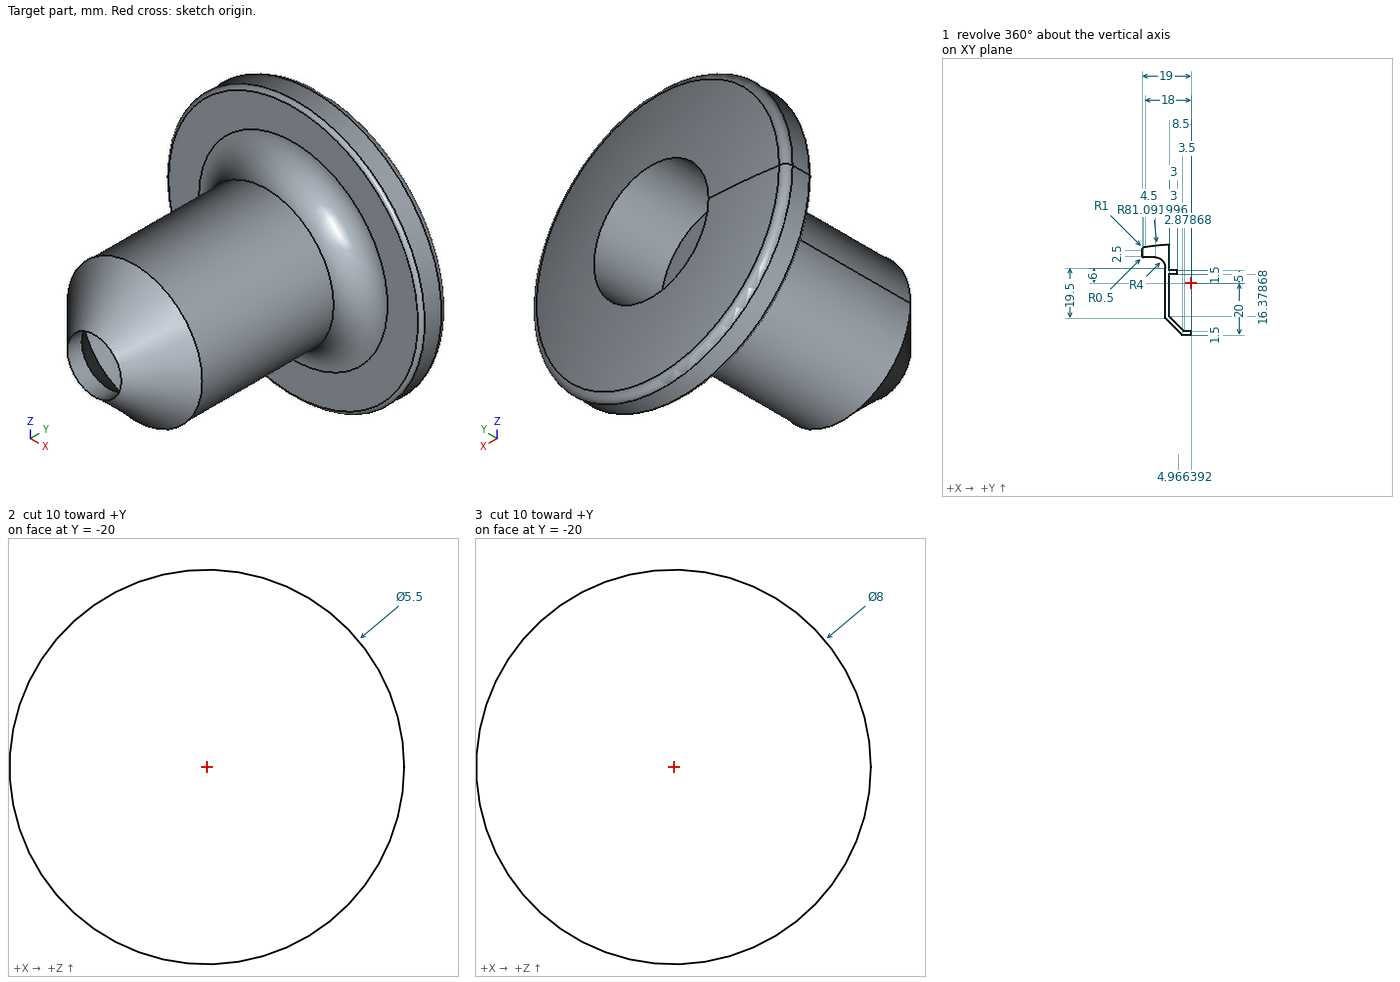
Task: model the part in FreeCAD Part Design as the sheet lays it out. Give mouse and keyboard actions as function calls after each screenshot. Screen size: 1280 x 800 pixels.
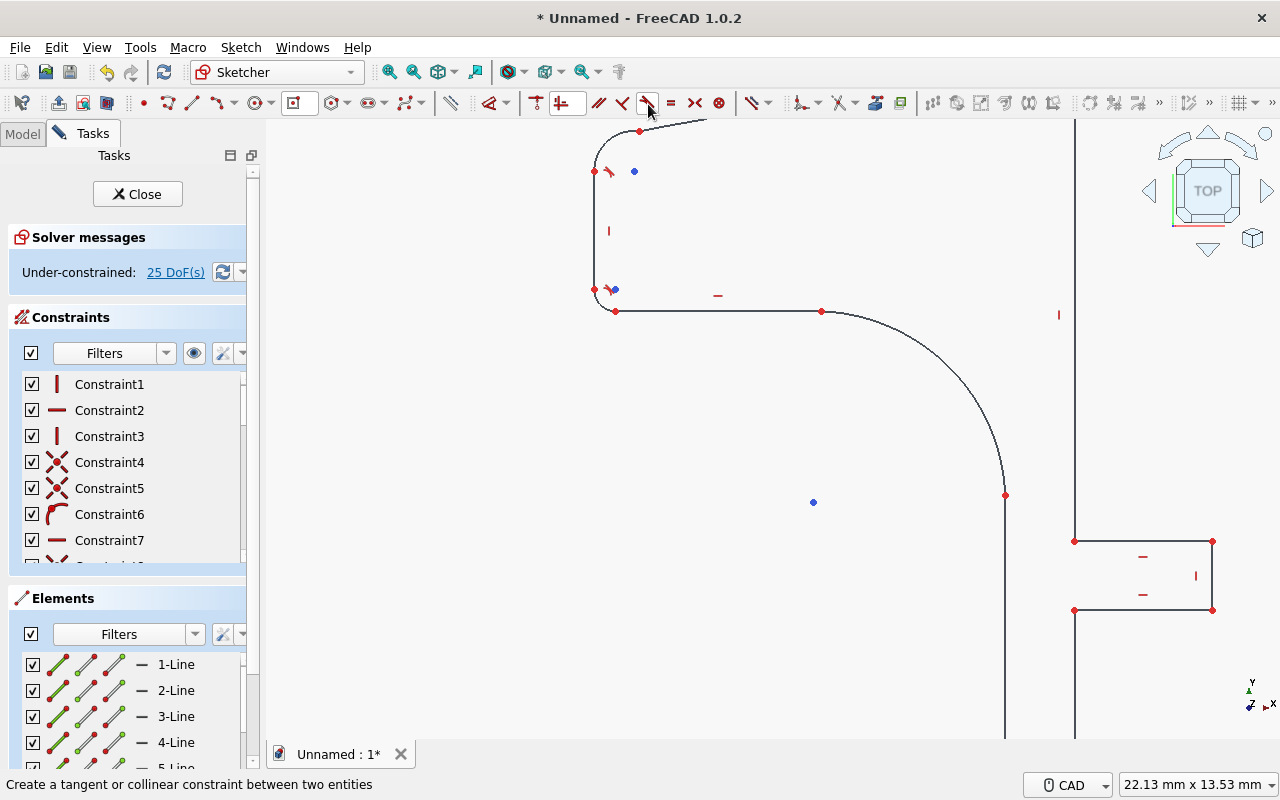
scroll(599, 280, down, 7)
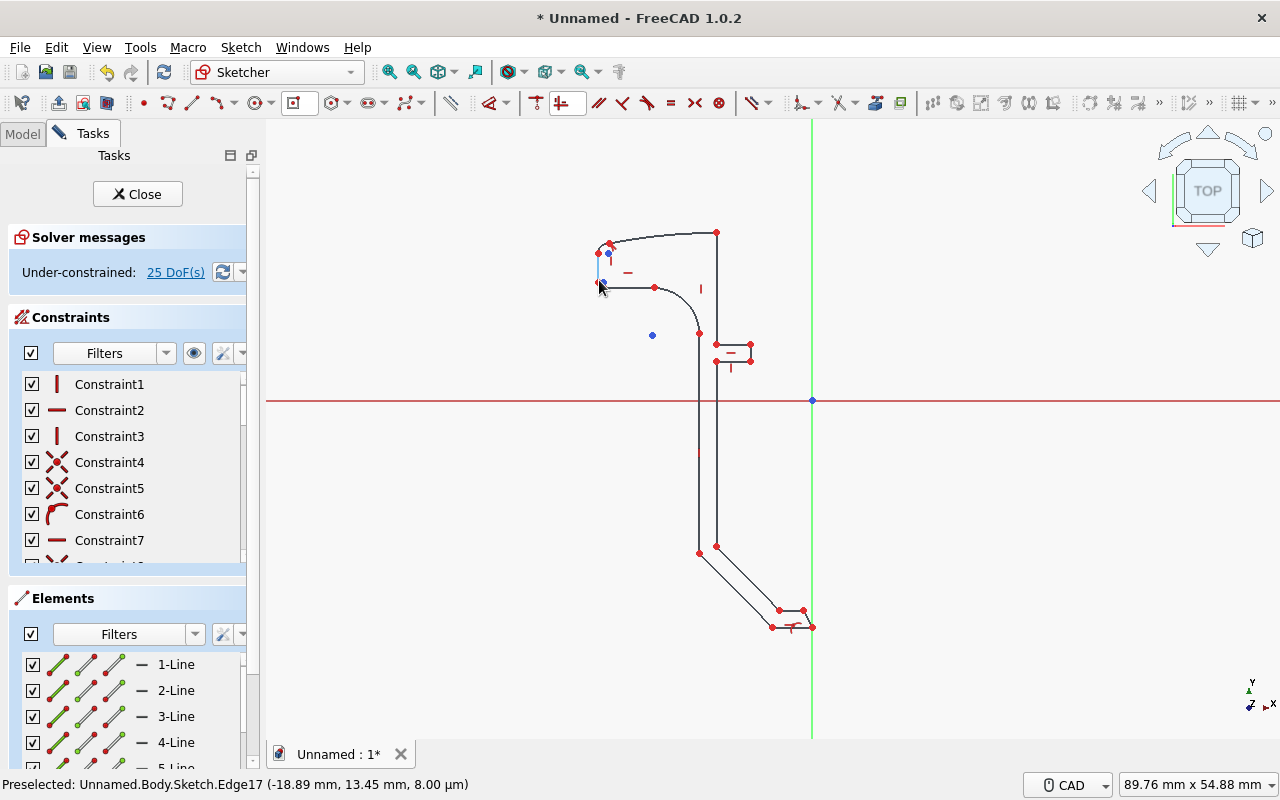
click(618, 288)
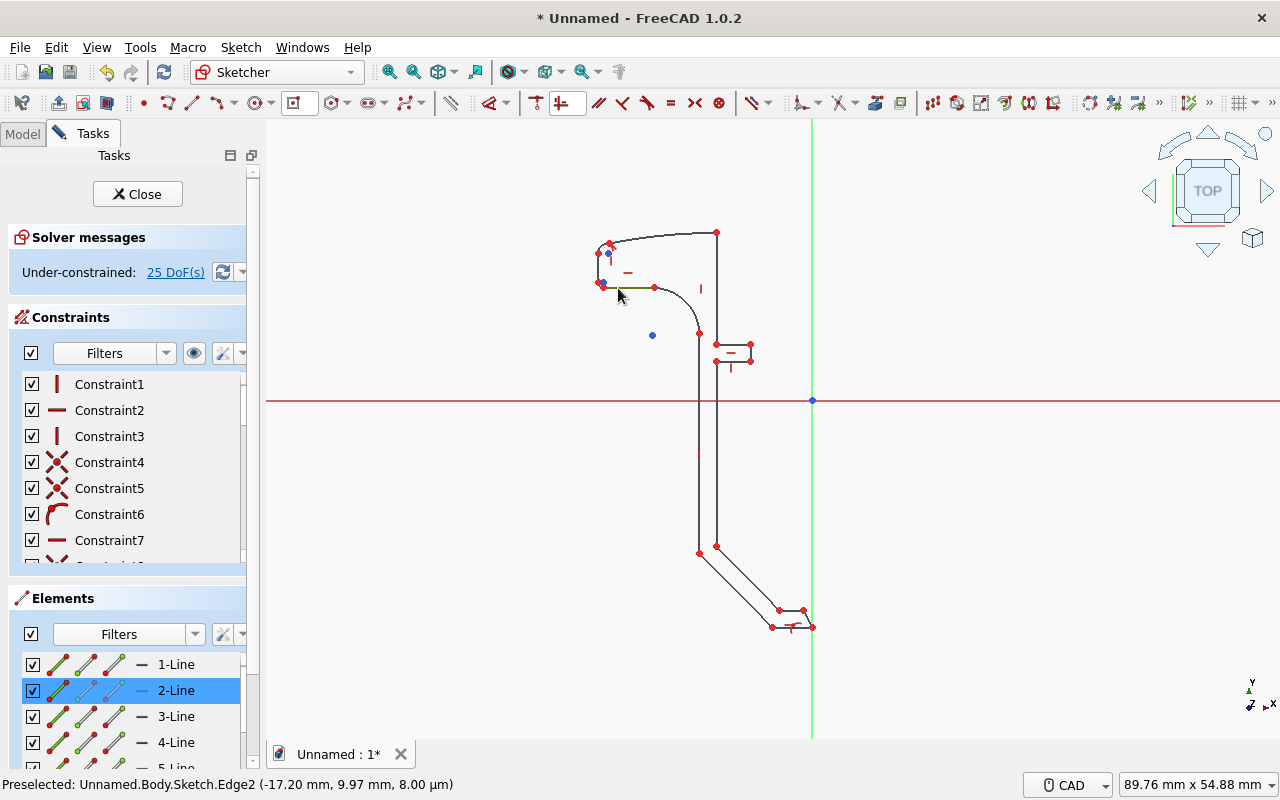
scroll(600, 286, up, 7)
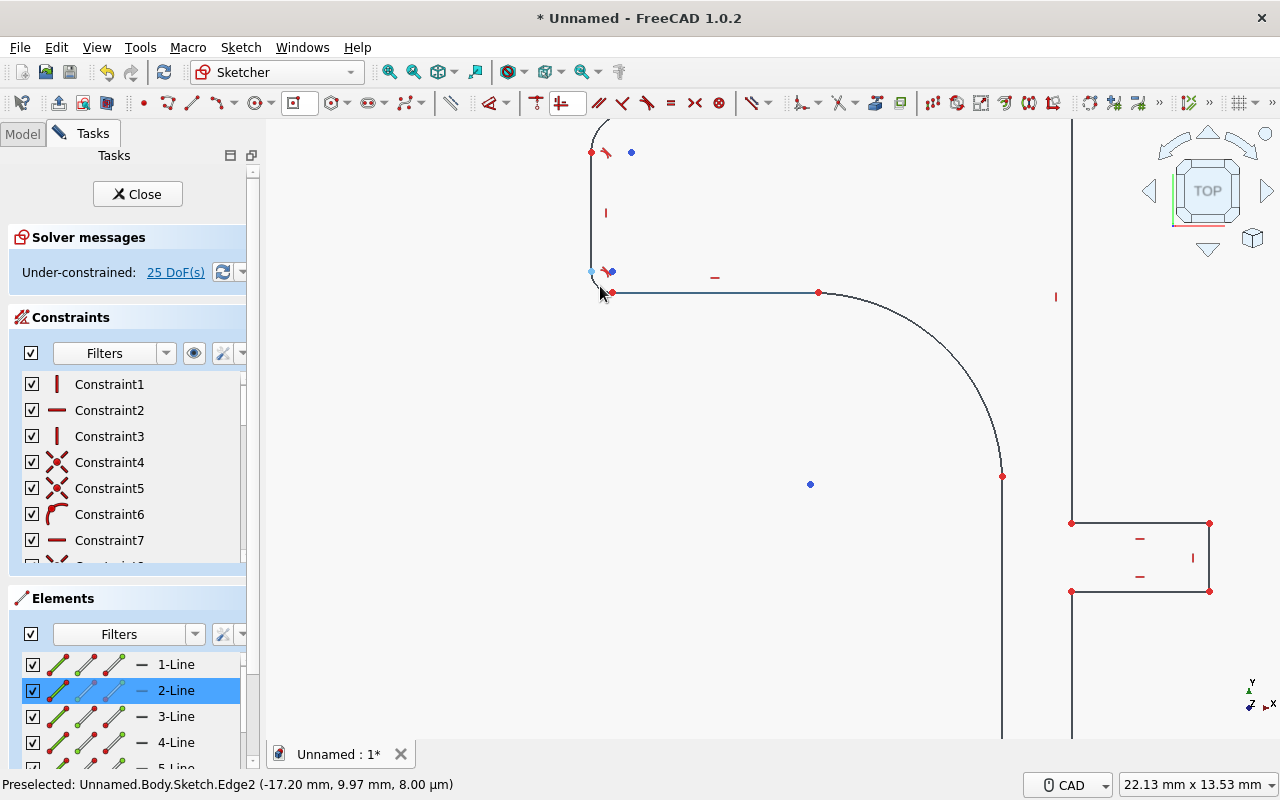
click(597, 286)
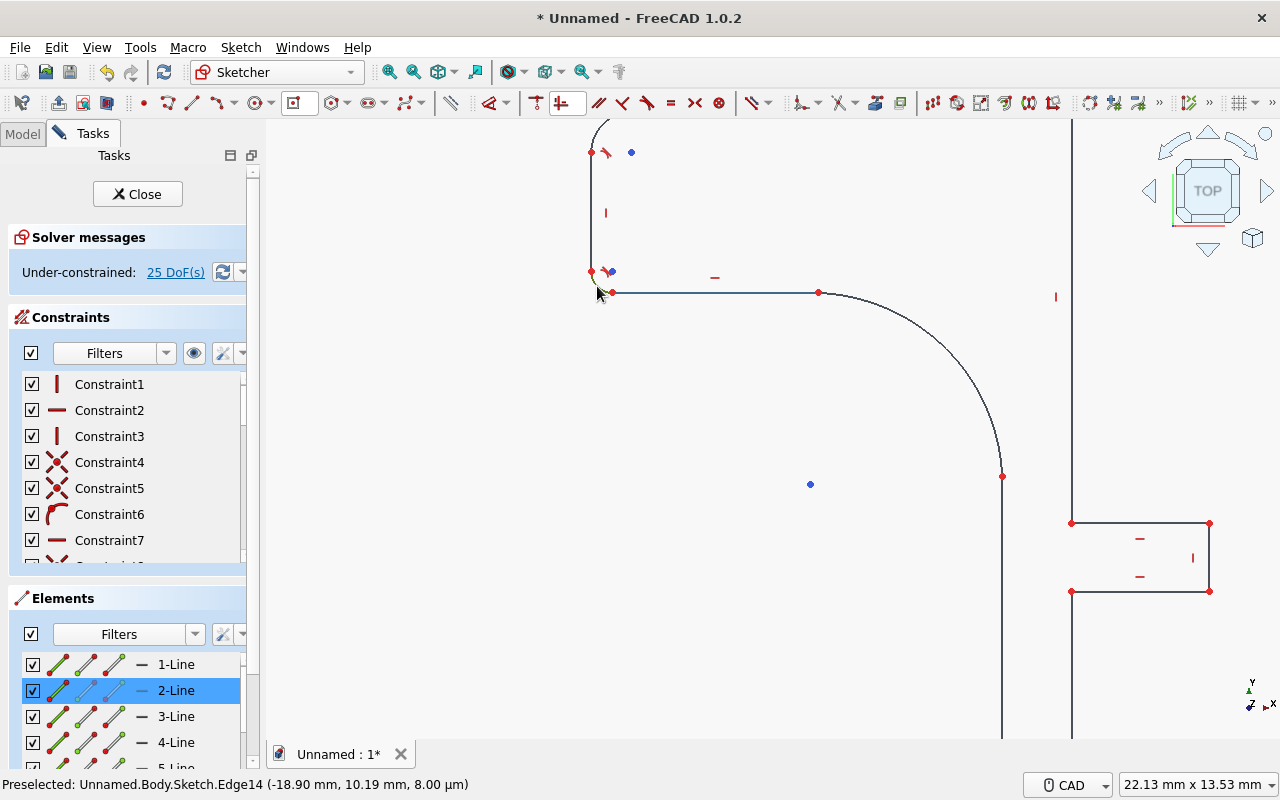
click(648, 104)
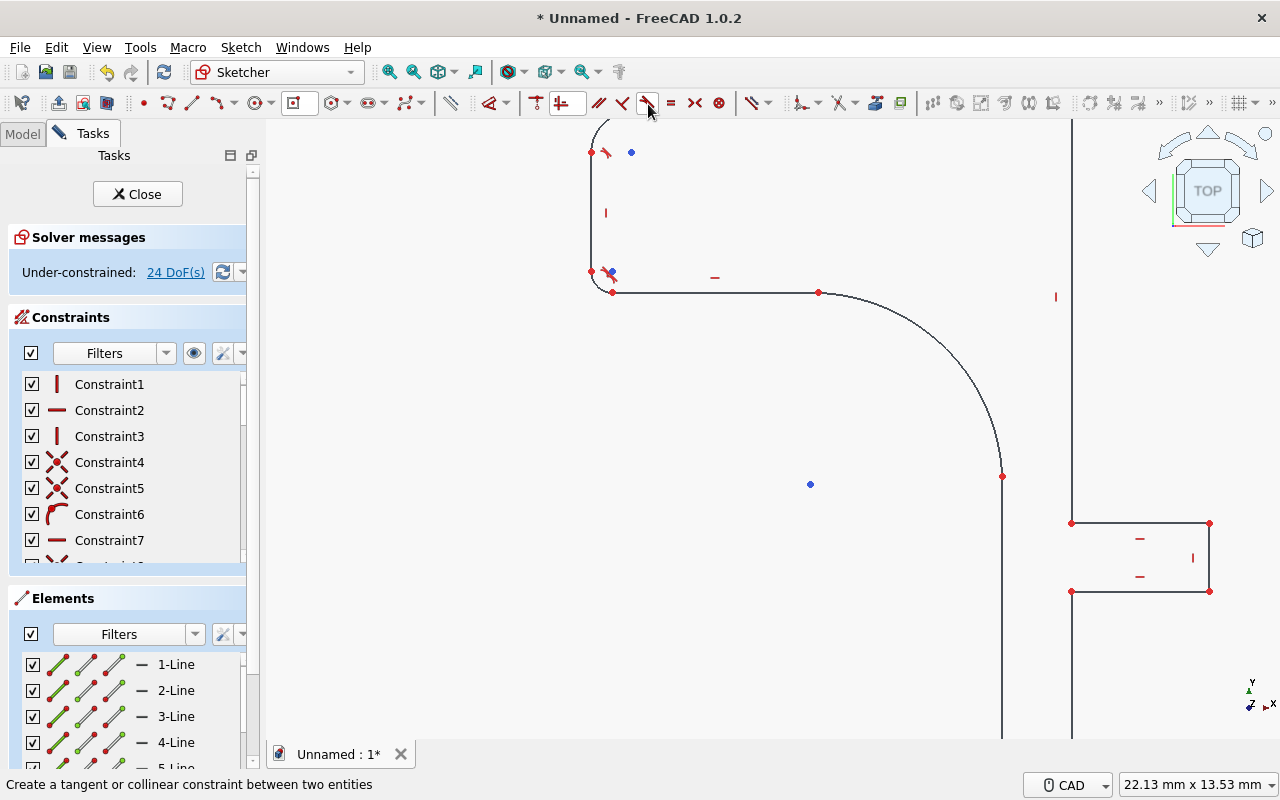
scroll(600, 286, down, 7)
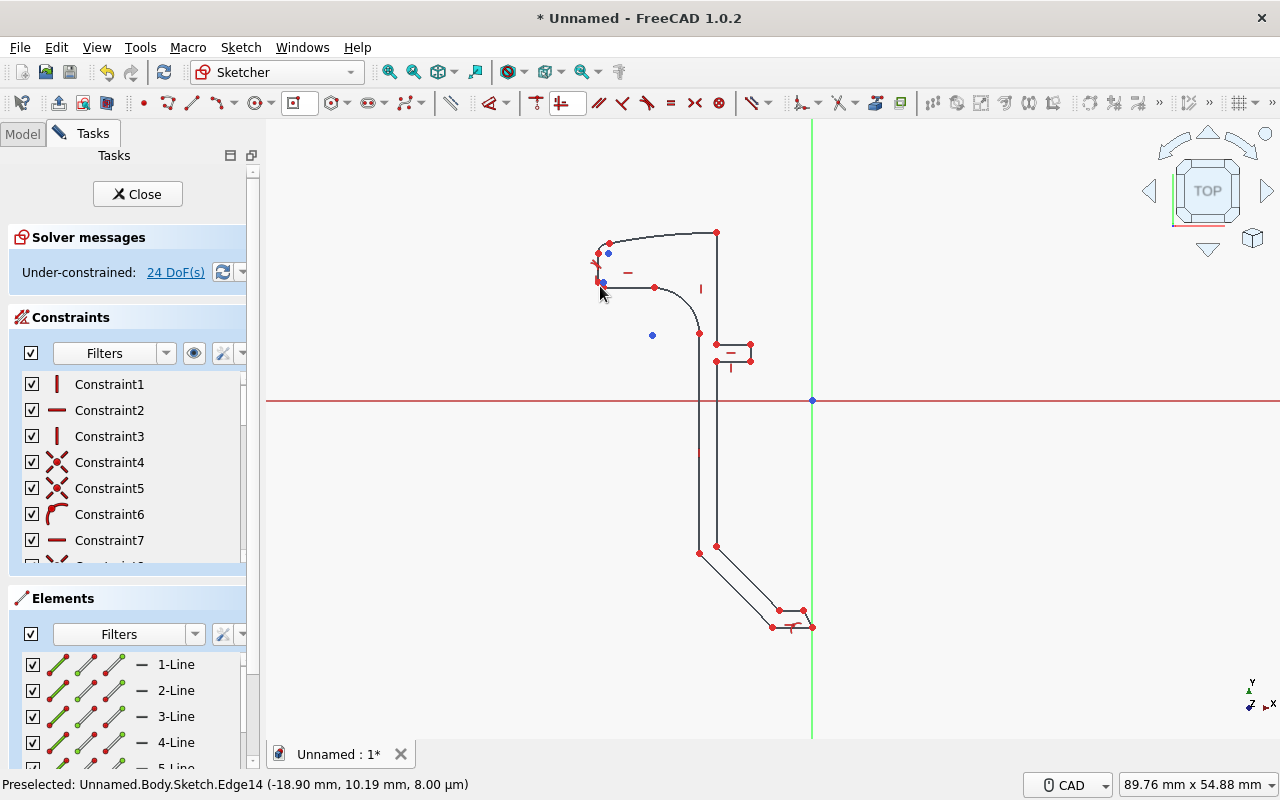
click(619, 288)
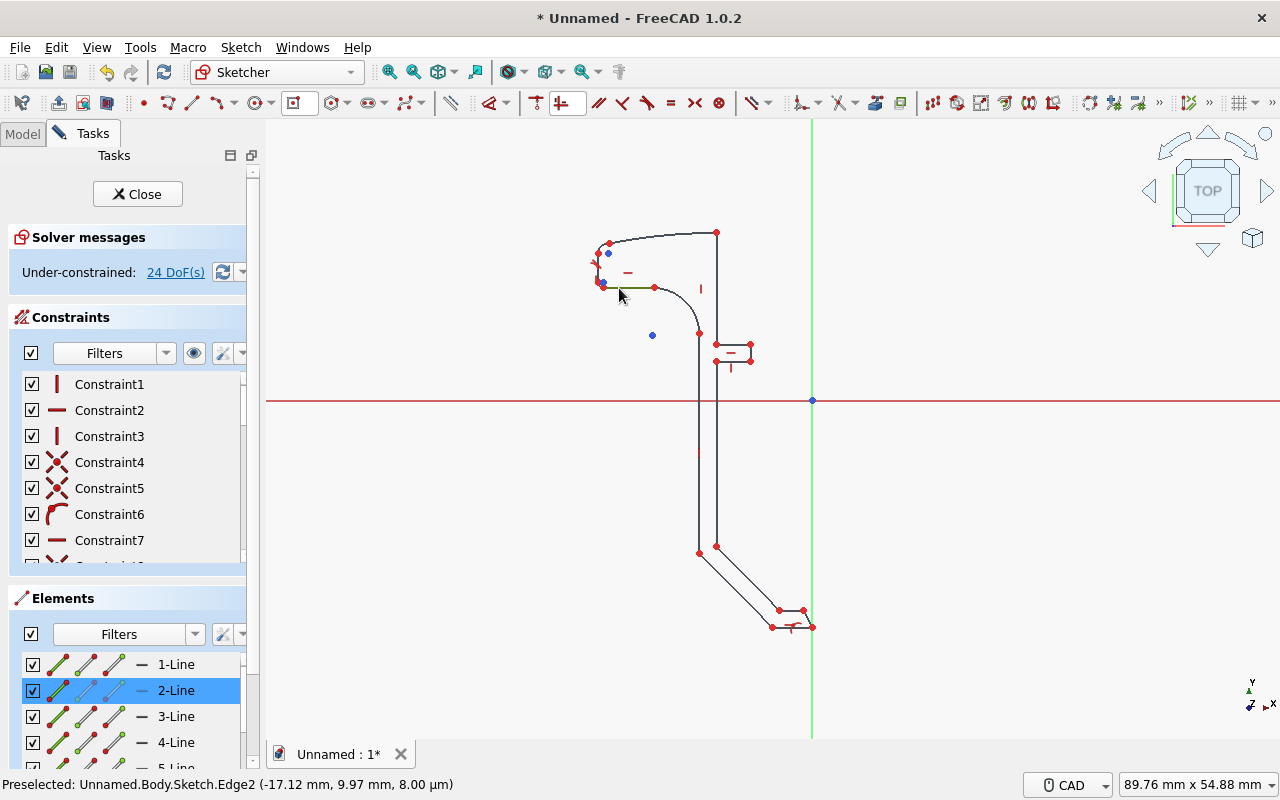
click(694, 313)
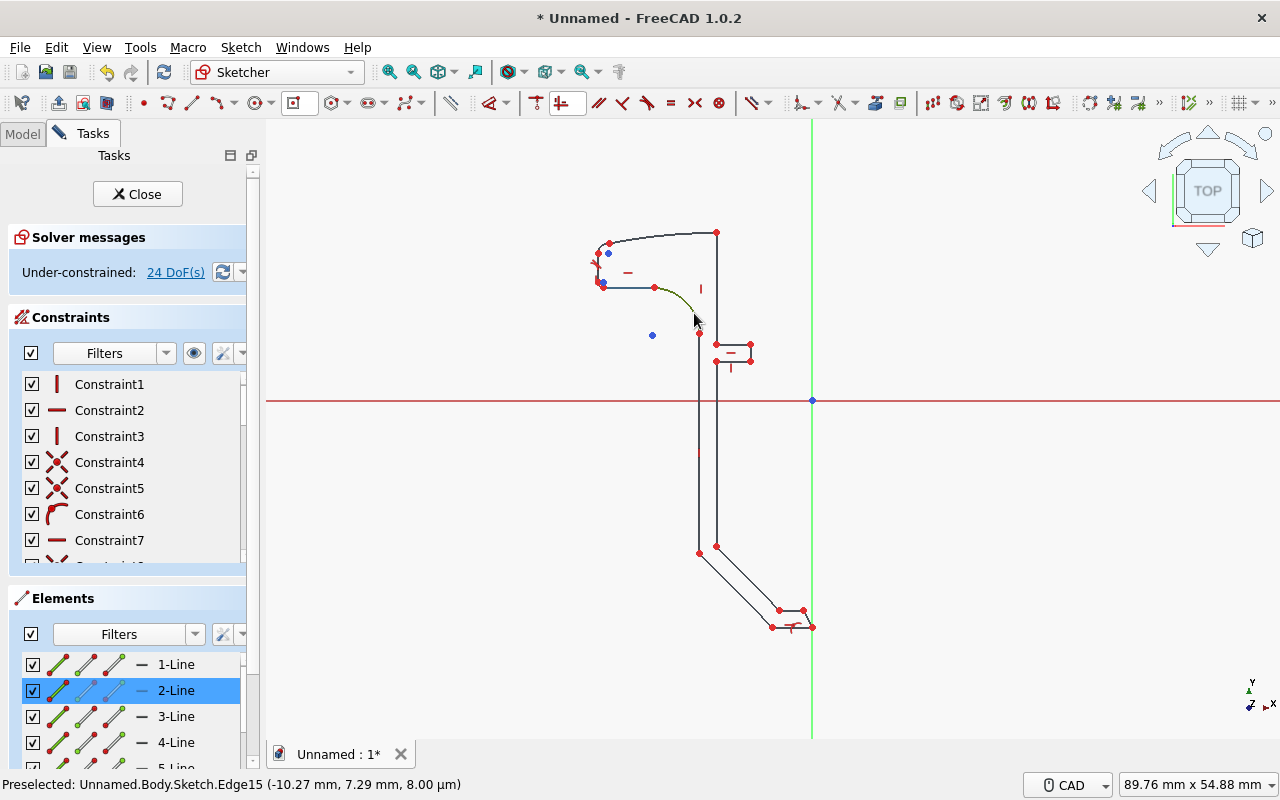
click(648, 104)